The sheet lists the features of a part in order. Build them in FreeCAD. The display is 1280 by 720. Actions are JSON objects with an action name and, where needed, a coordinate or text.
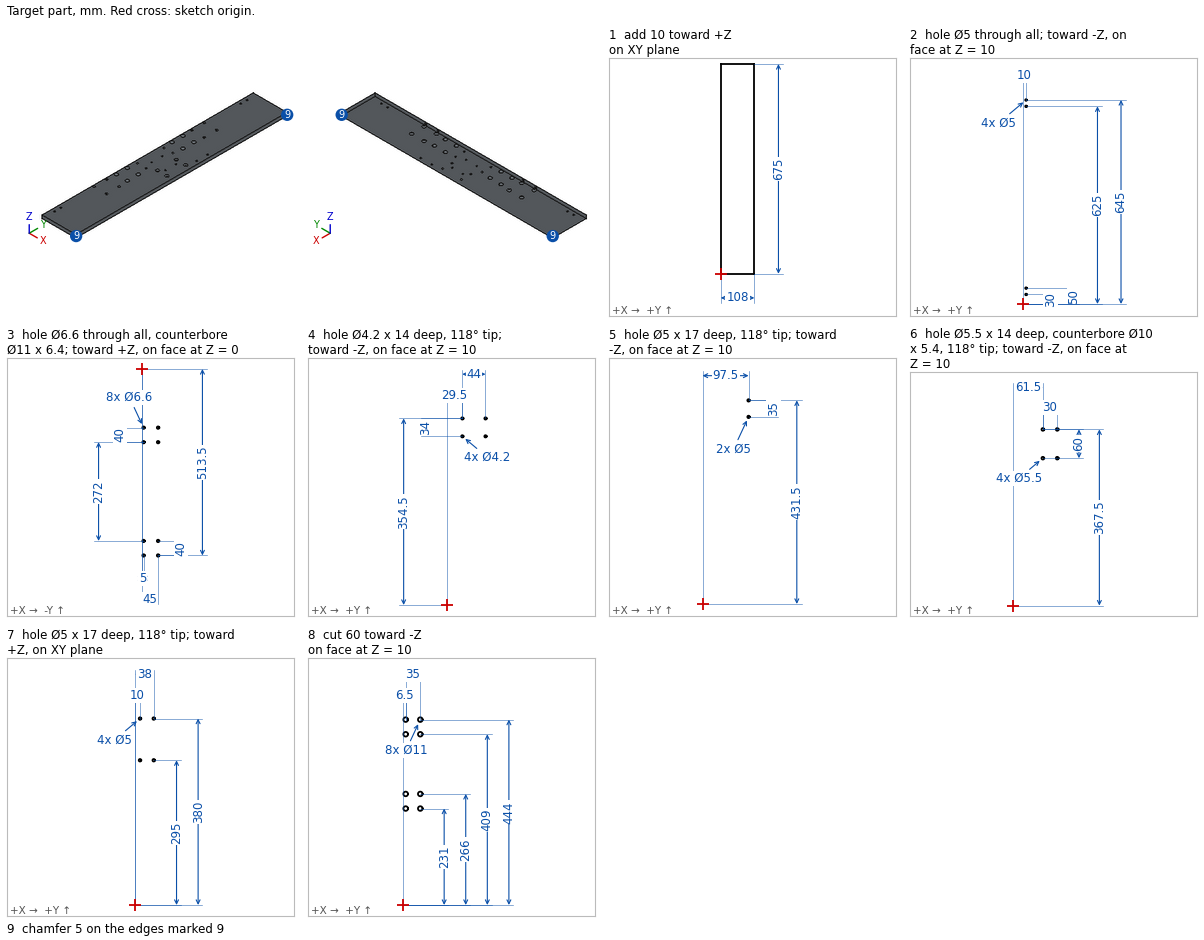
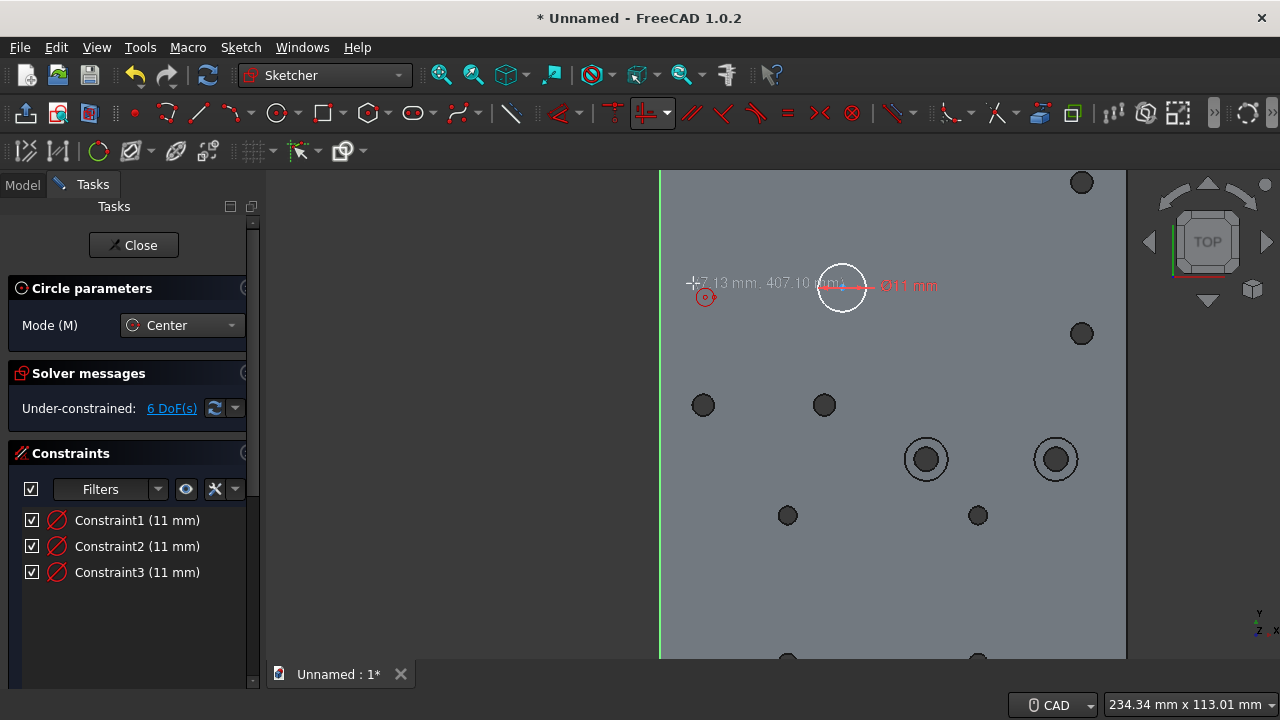
{"action": "left_click", "coordinate": [688, 280]}
{"action": "mouse_move", "coordinate": [705, 263]}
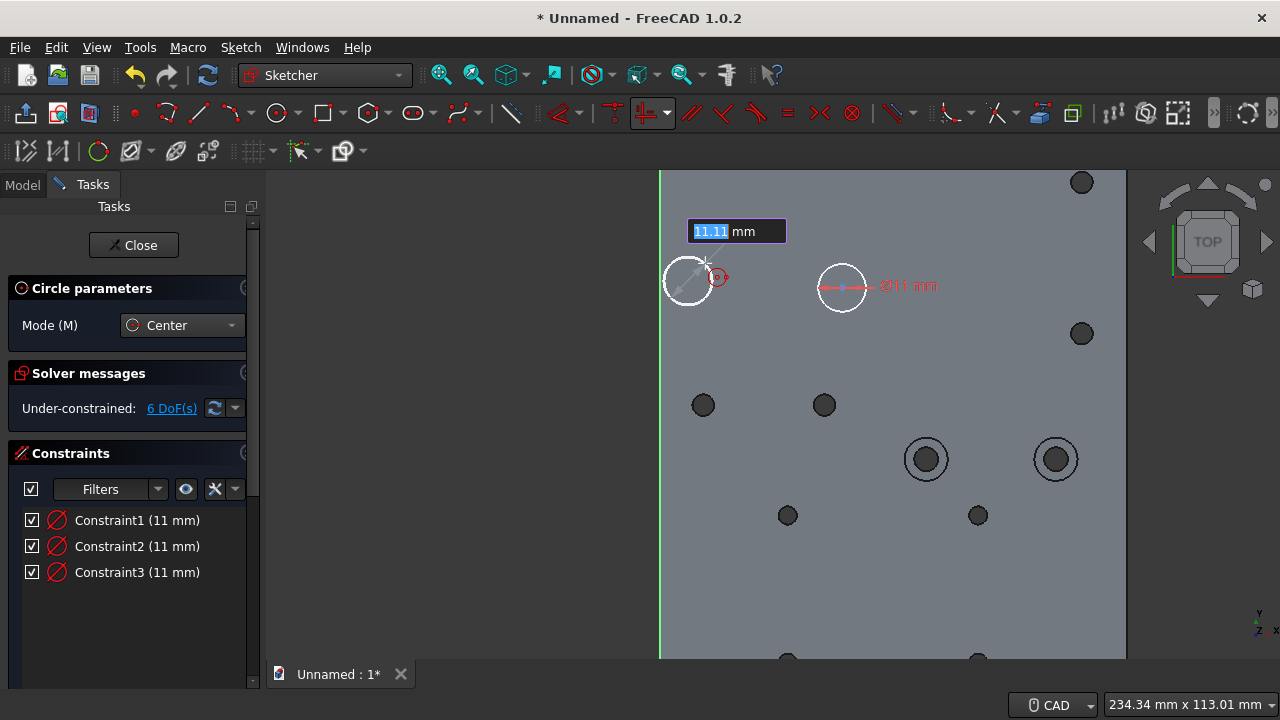
{"action": "type", "text": "11"}
{"action": "key", "text": "Return"}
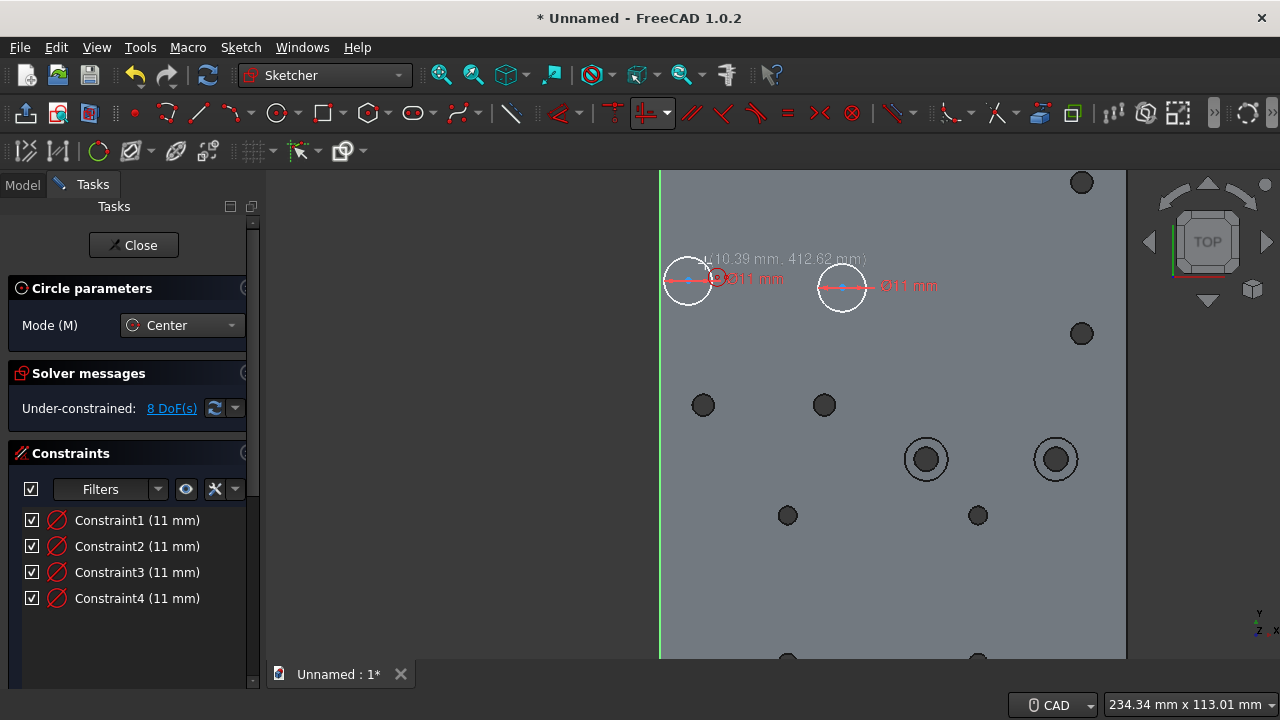
{"action": "scroll", "coordinate": [693, 283], "scroll_direction": "down", "scroll_amount": 9}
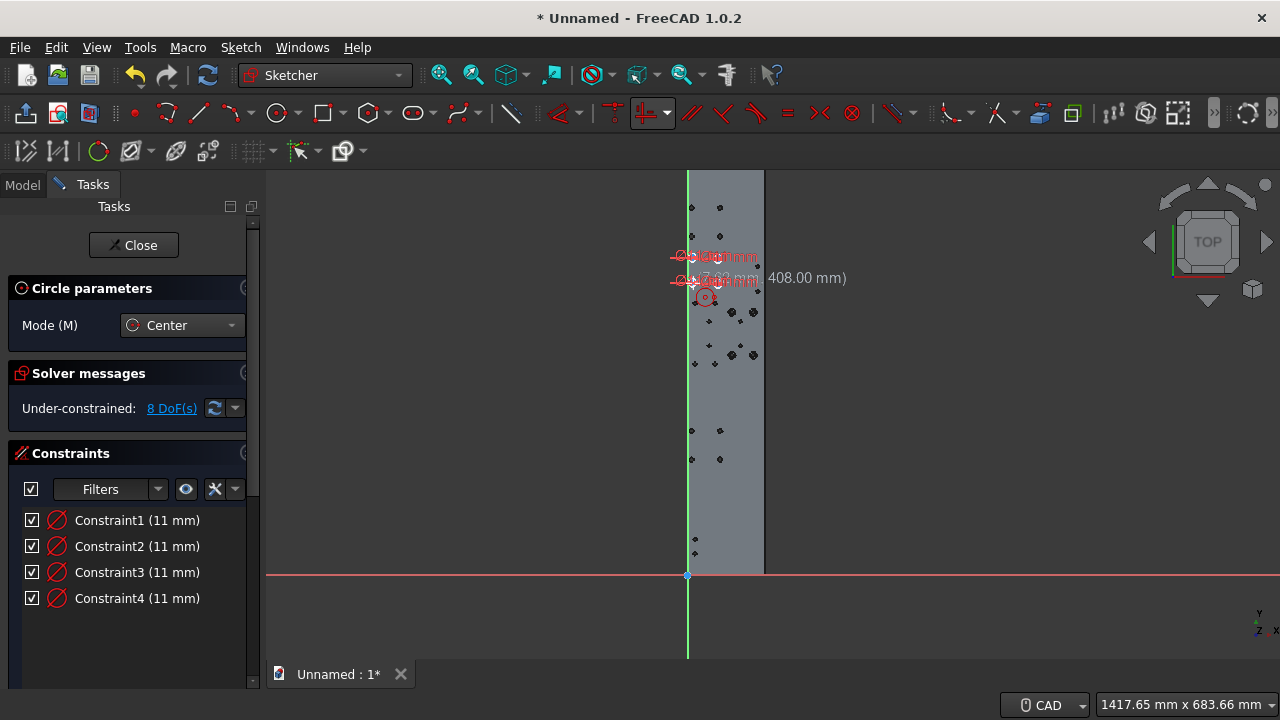
{"action": "scroll", "coordinate": [718, 385], "scroll_direction": "up", "scroll_amount": 9}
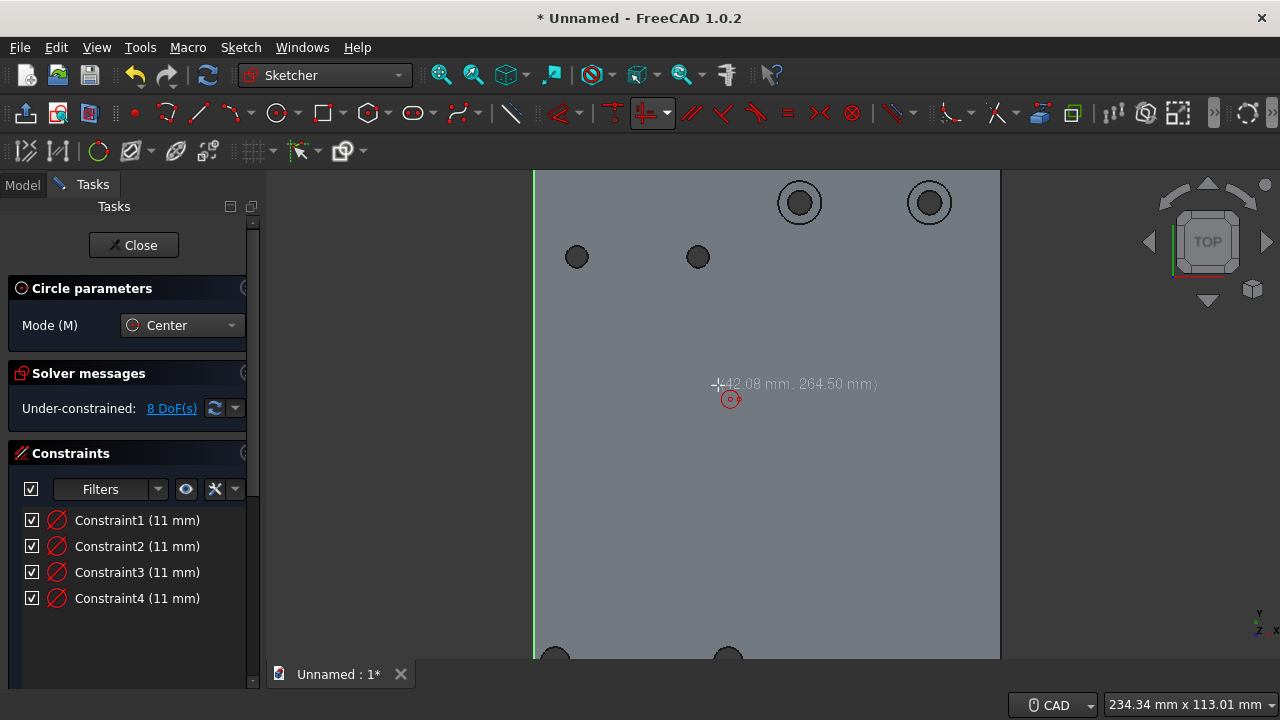
{"action": "scroll", "coordinate": [718, 386], "scroll_direction": "down", "scroll_amount": 9}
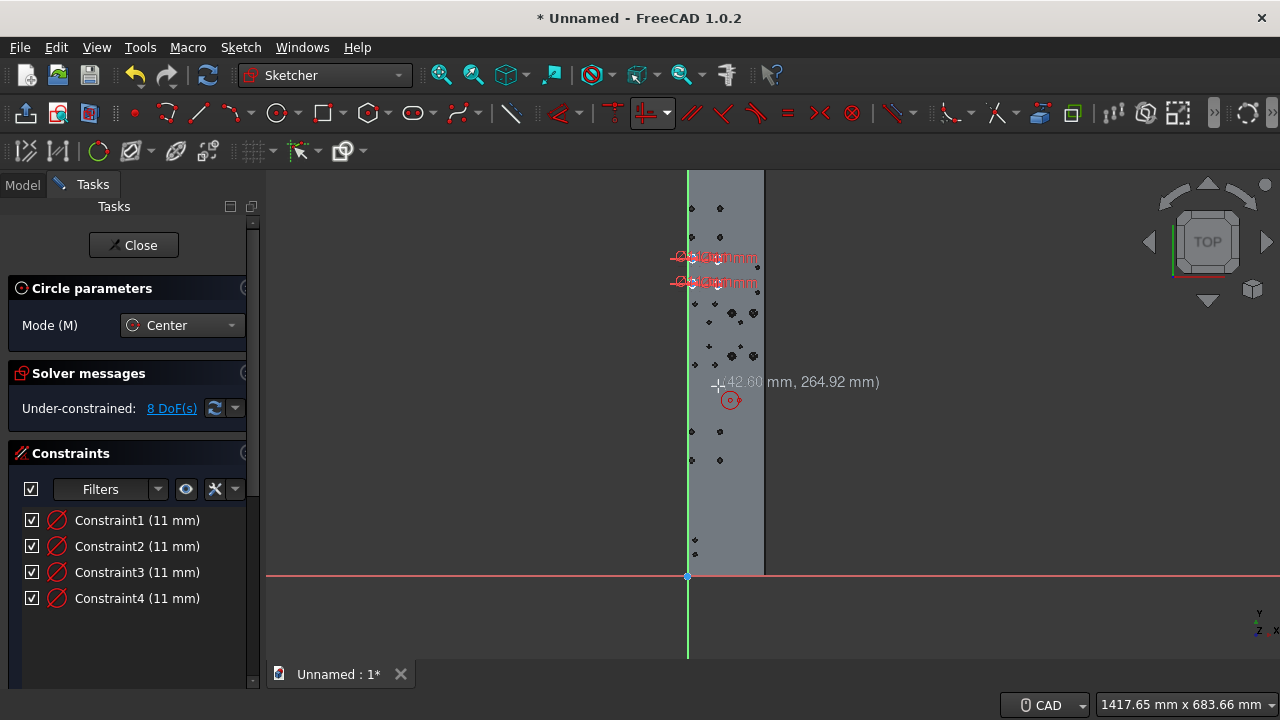
{"action": "left_click", "coordinate": [718, 386]}
{"action": "mouse_move", "coordinate": [720, 383]}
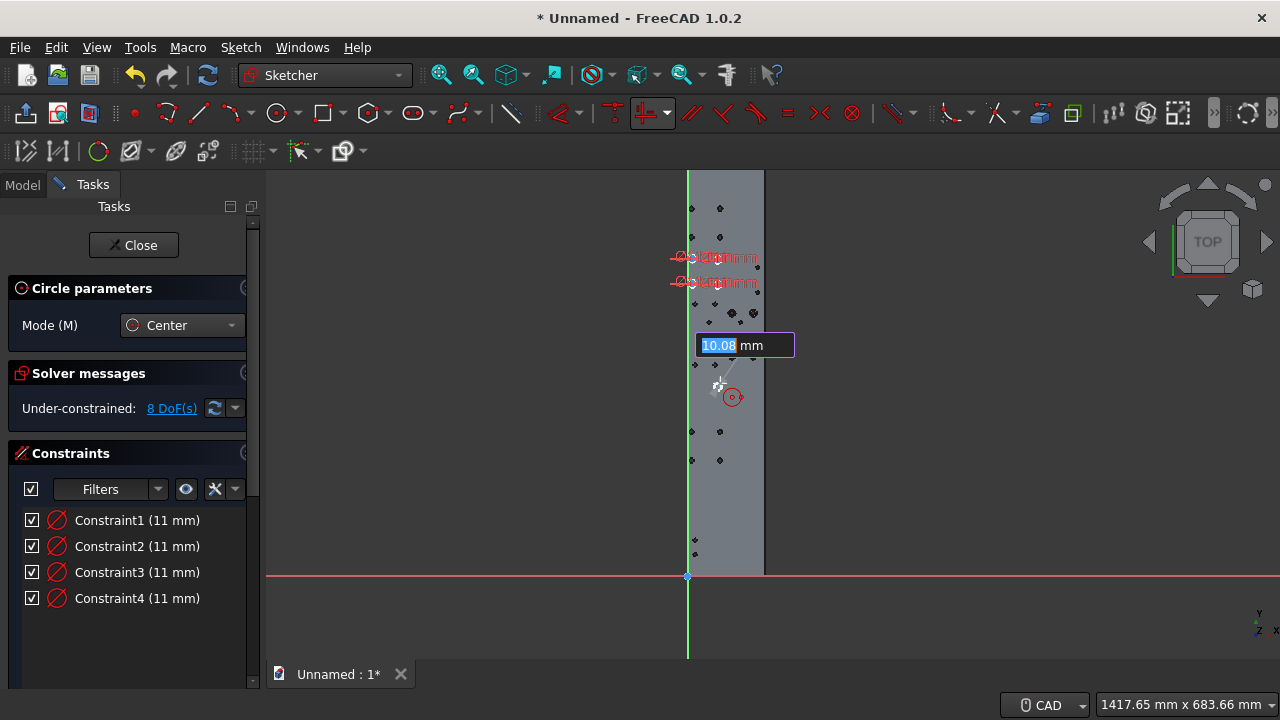
{"action": "type", "text": "11"}
{"action": "key", "text": "Return"}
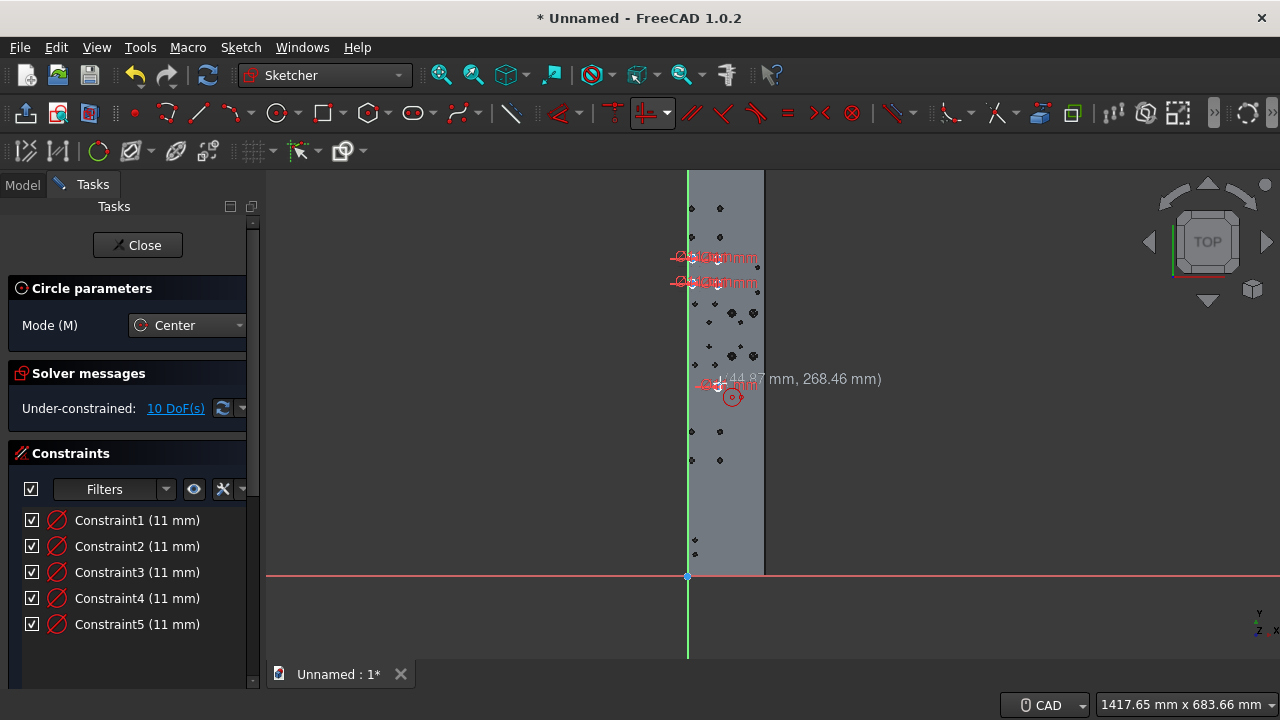
{"action": "scroll", "coordinate": [718, 411], "scroll_direction": "up", "scroll_amount": 9}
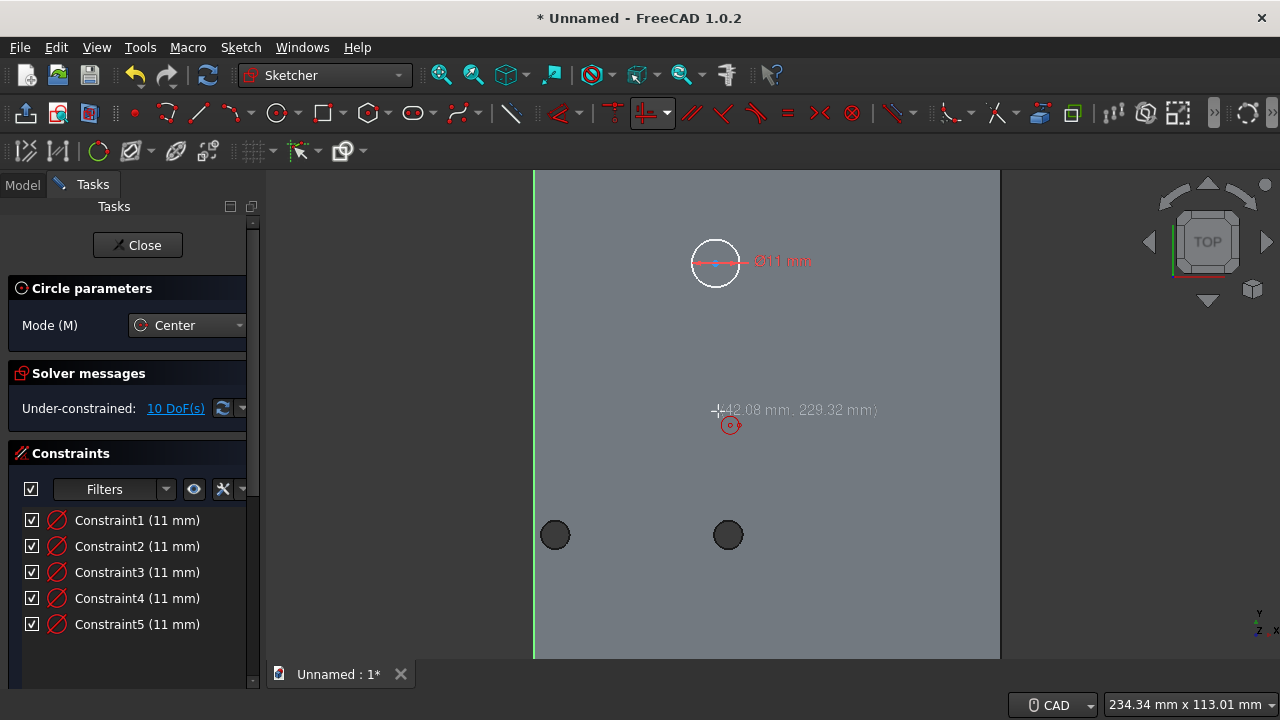
{"action": "scroll", "coordinate": [718, 411], "scroll_direction": "down", "scroll_amount": 9}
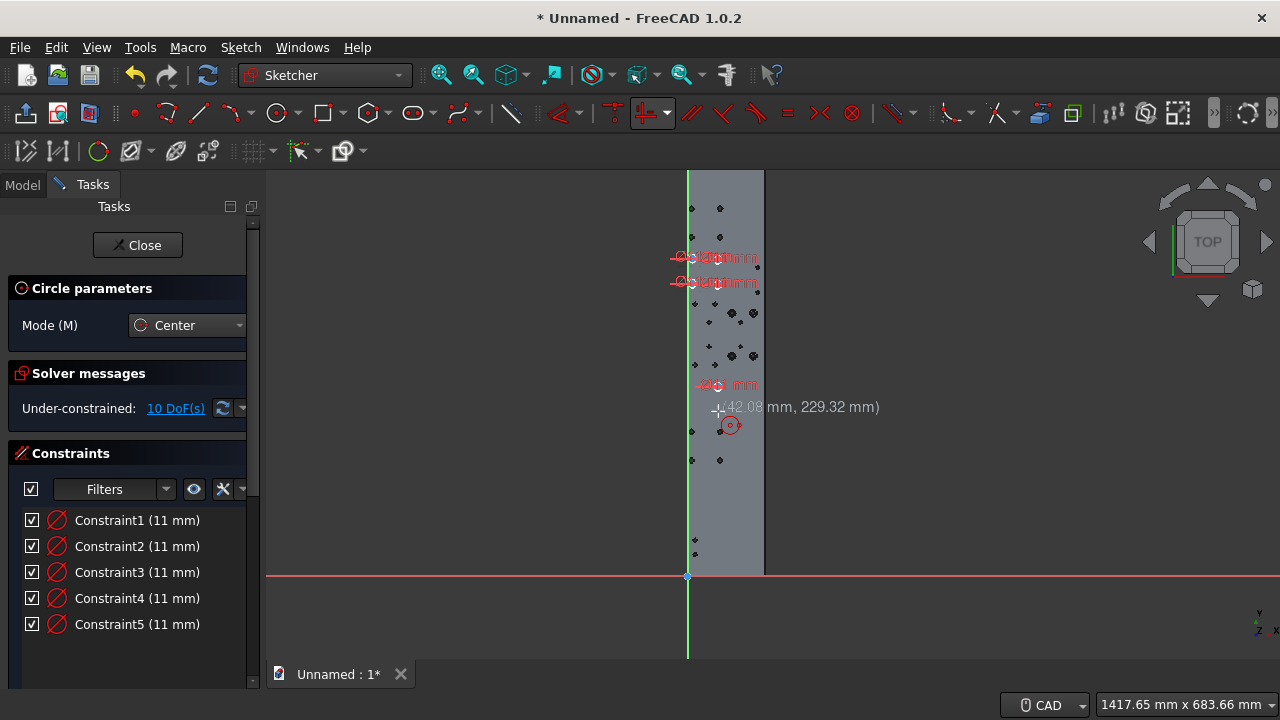
{"action": "left_click", "coordinate": [718, 411]}
{"action": "mouse_move", "coordinate": [720, 408]}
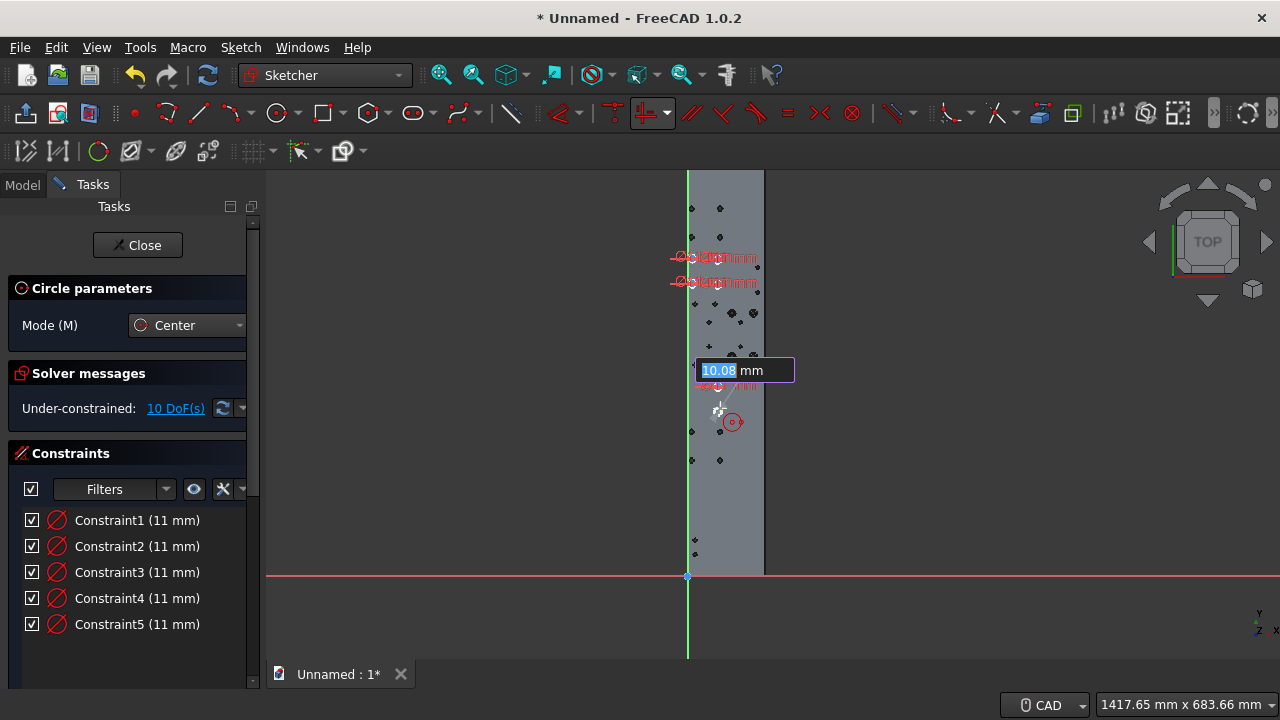
{"action": "type", "text": "11"}
{"action": "key", "text": "Return"}